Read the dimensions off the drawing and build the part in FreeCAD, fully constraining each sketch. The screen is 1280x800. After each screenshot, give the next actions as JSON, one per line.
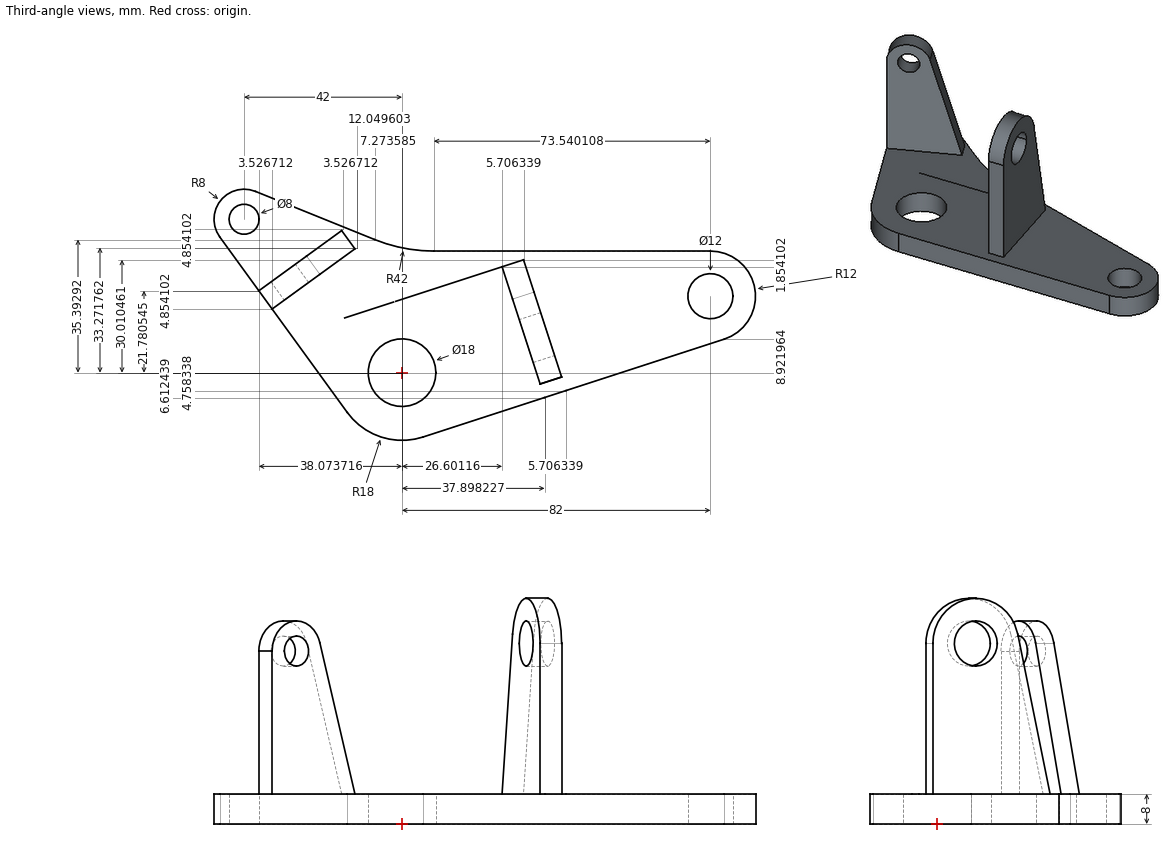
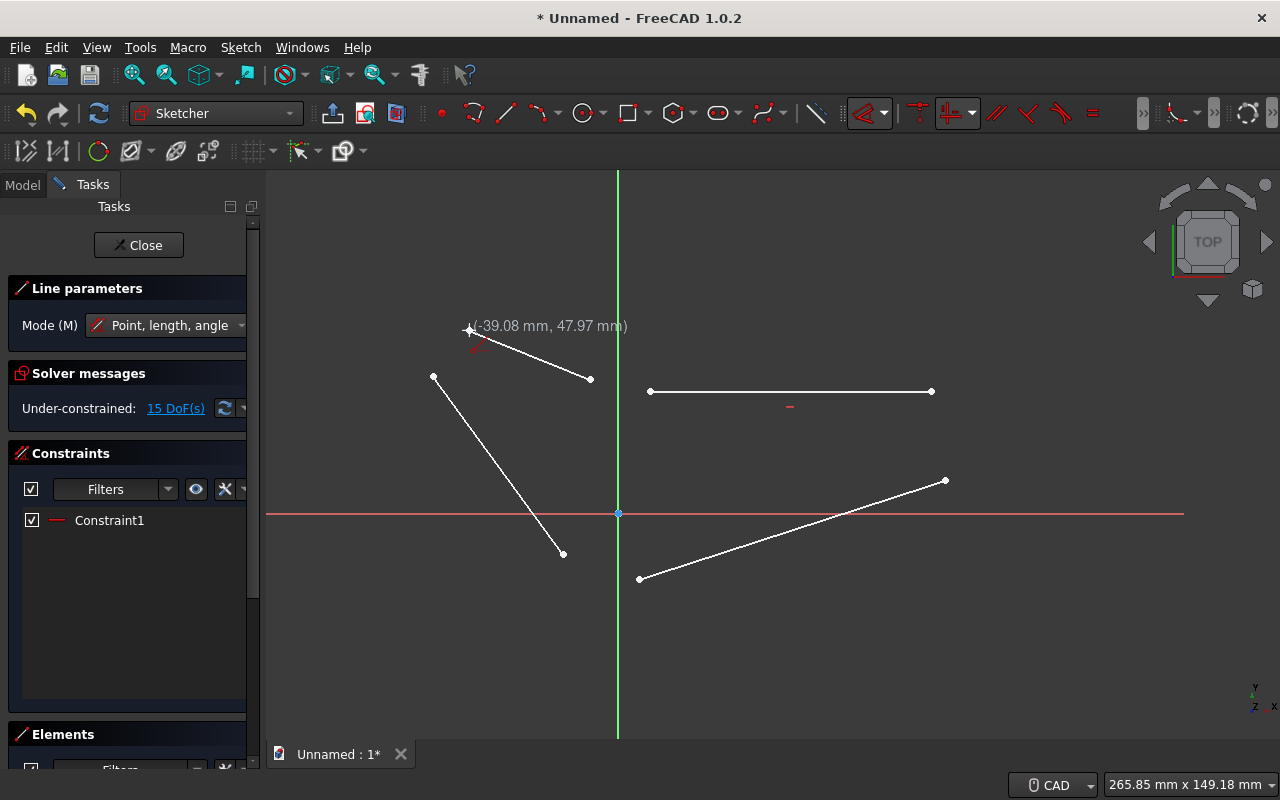
{"action": "key", "text": "g 3 a"}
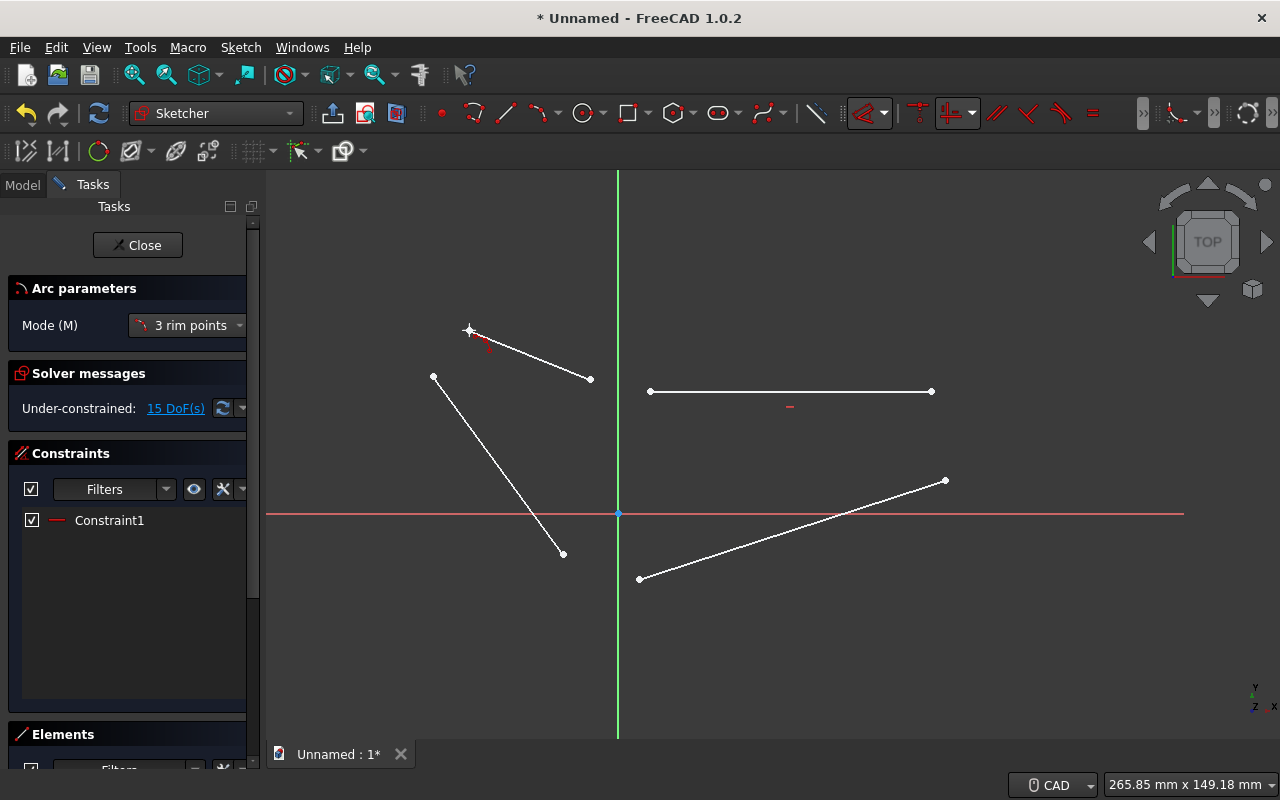
{"action": "left_click", "coordinate": [563, 555]}
{"action": "left_click", "coordinate": [639, 580]}
{"action": "left_click", "coordinate": [597, 579]}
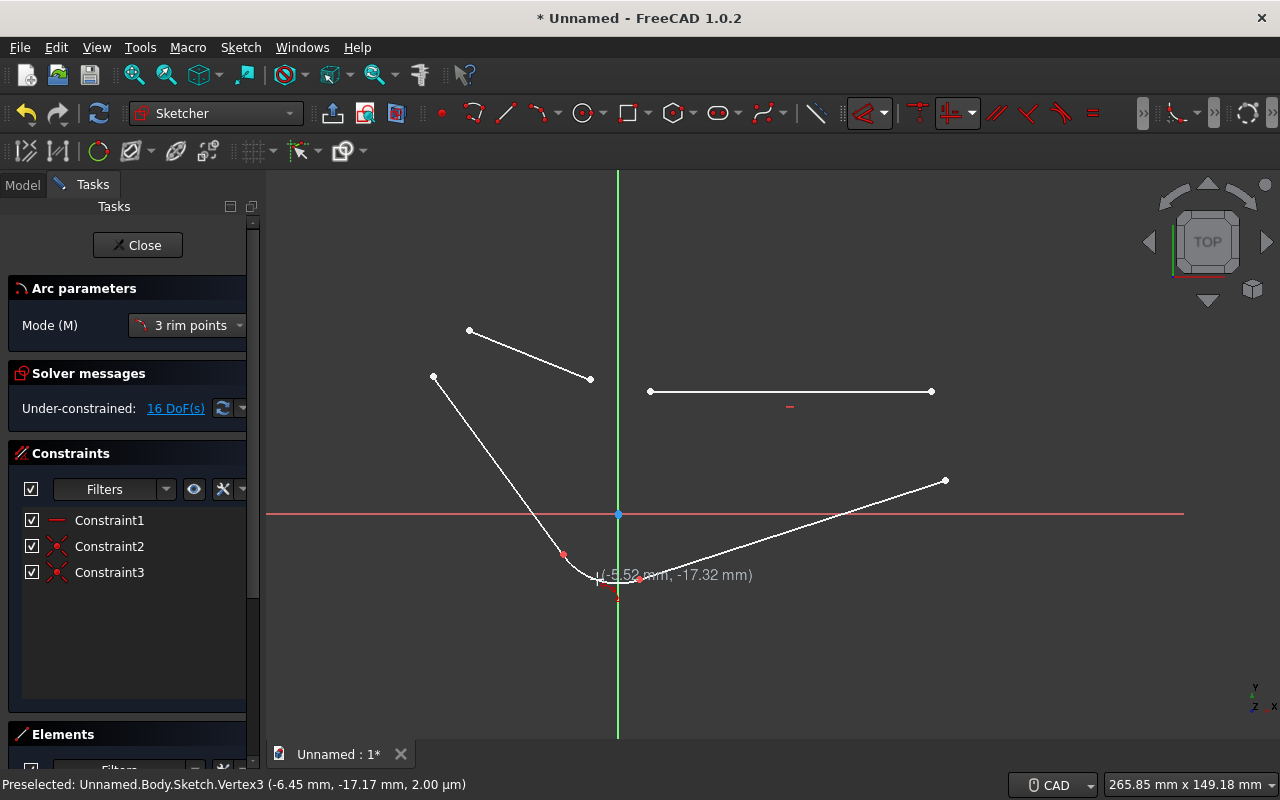
{"action": "left_click", "coordinate": [945, 481]}
{"action": "left_click", "coordinate": [931, 392]}
{"action": "left_click", "coordinate": [976, 429]}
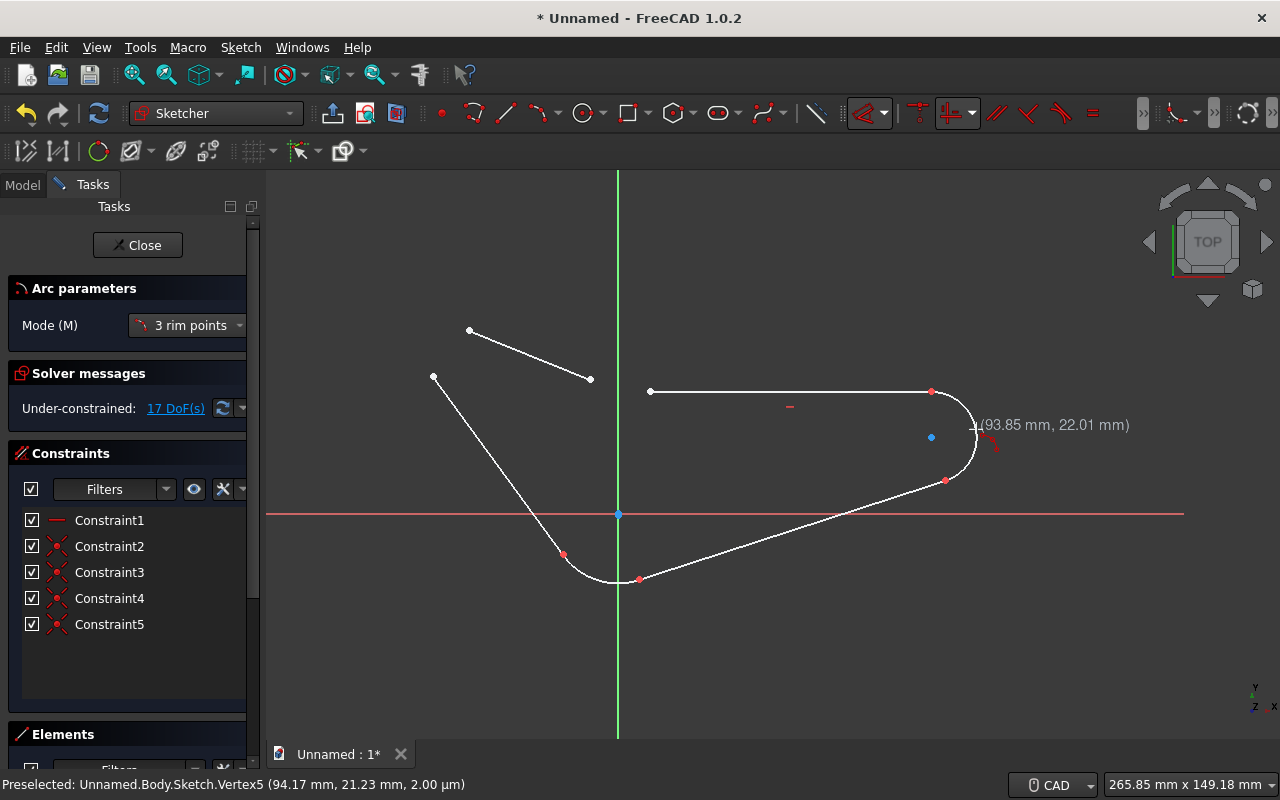
{"action": "left_click", "coordinate": [650, 392]}
{"action": "left_click", "coordinate": [590, 380]}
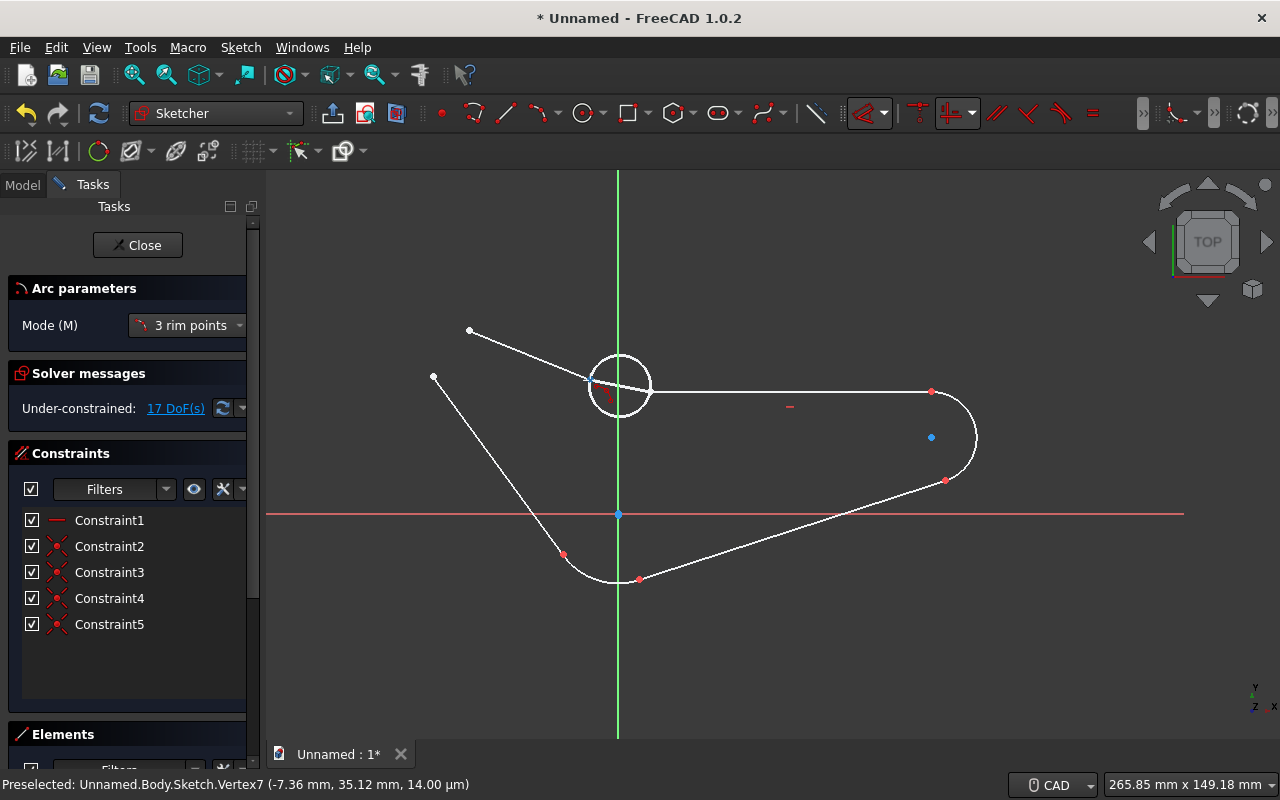
{"action": "scroll", "coordinate": [626, 389], "scroll_direction": "up", "scroll_amount": 9}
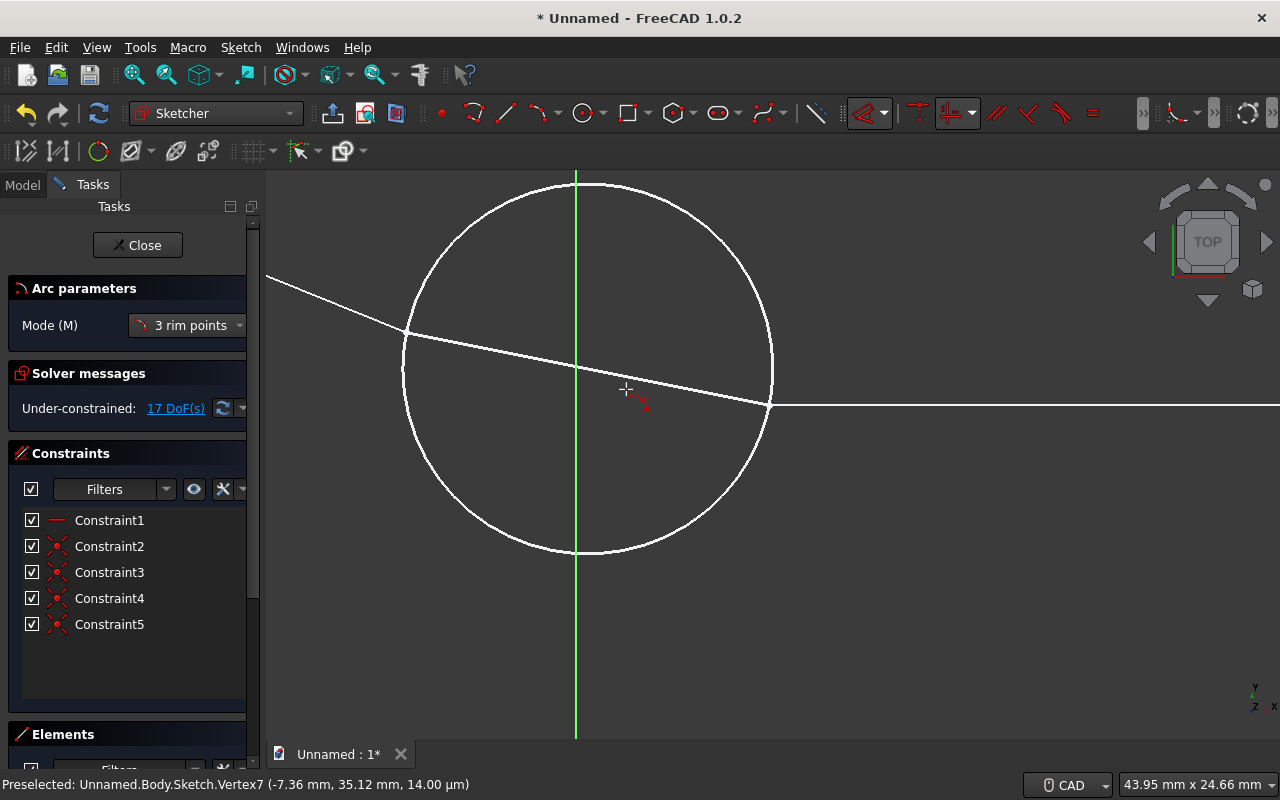
{"action": "left_click", "coordinate": [623, 385]}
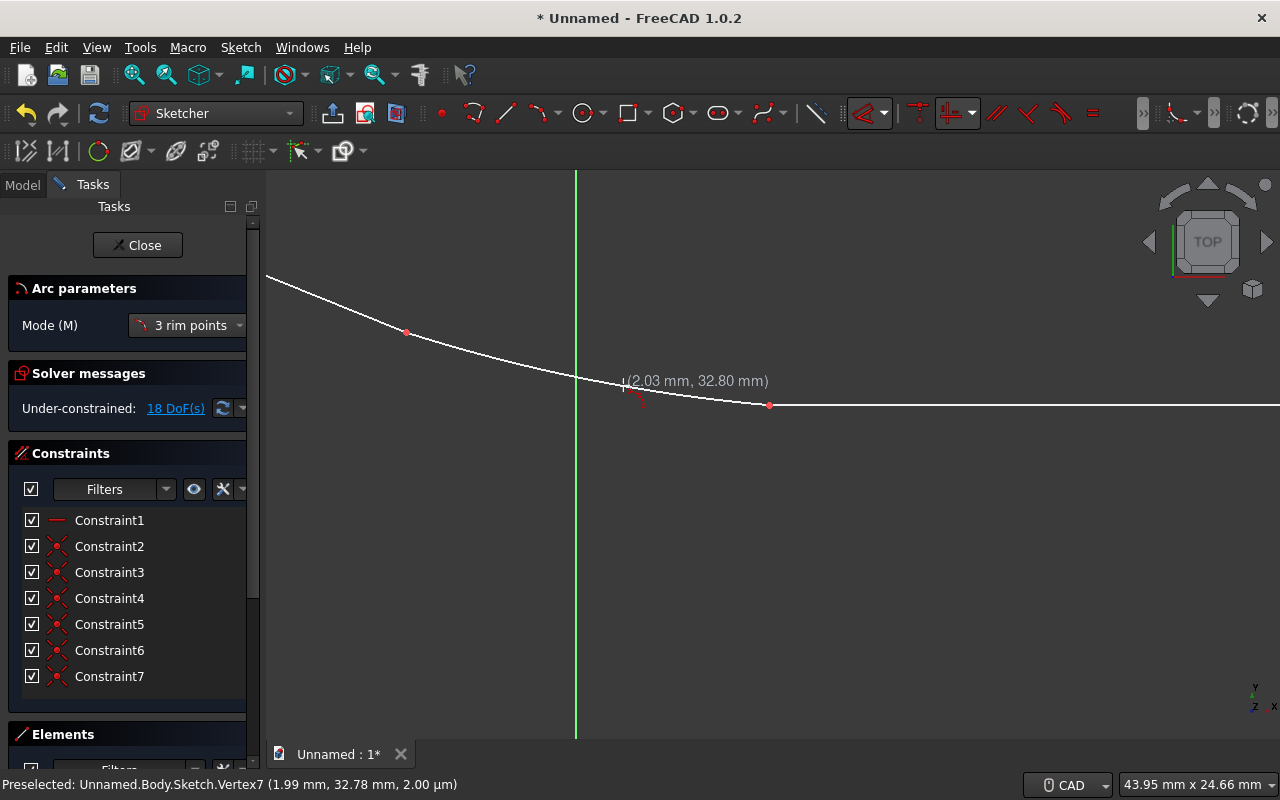
{"action": "scroll", "coordinate": [626, 389], "scroll_direction": "down", "scroll_amount": 9}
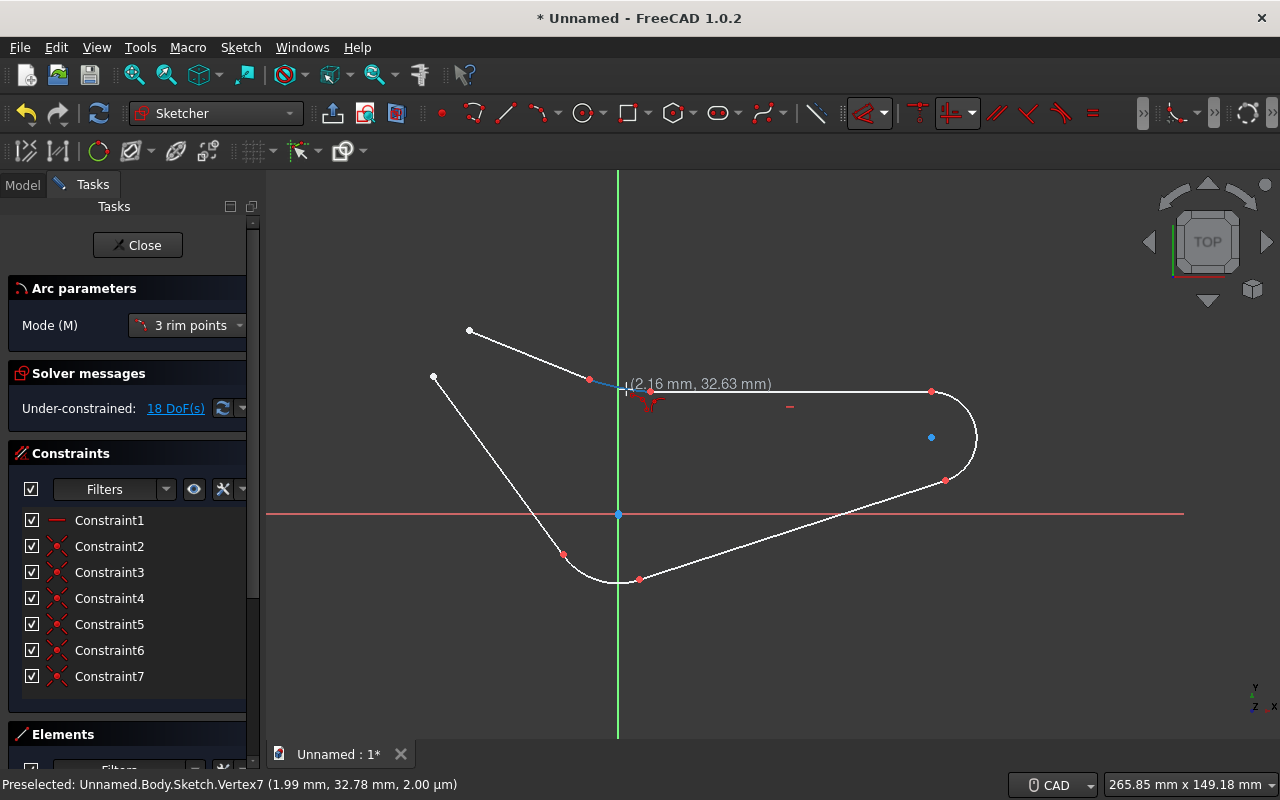
{"action": "left_click", "coordinate": [469, 331]}
{"action": "left_click", "coordinate": [433, 377]}
{"action": "left_click", "coordinate": [434, 340]}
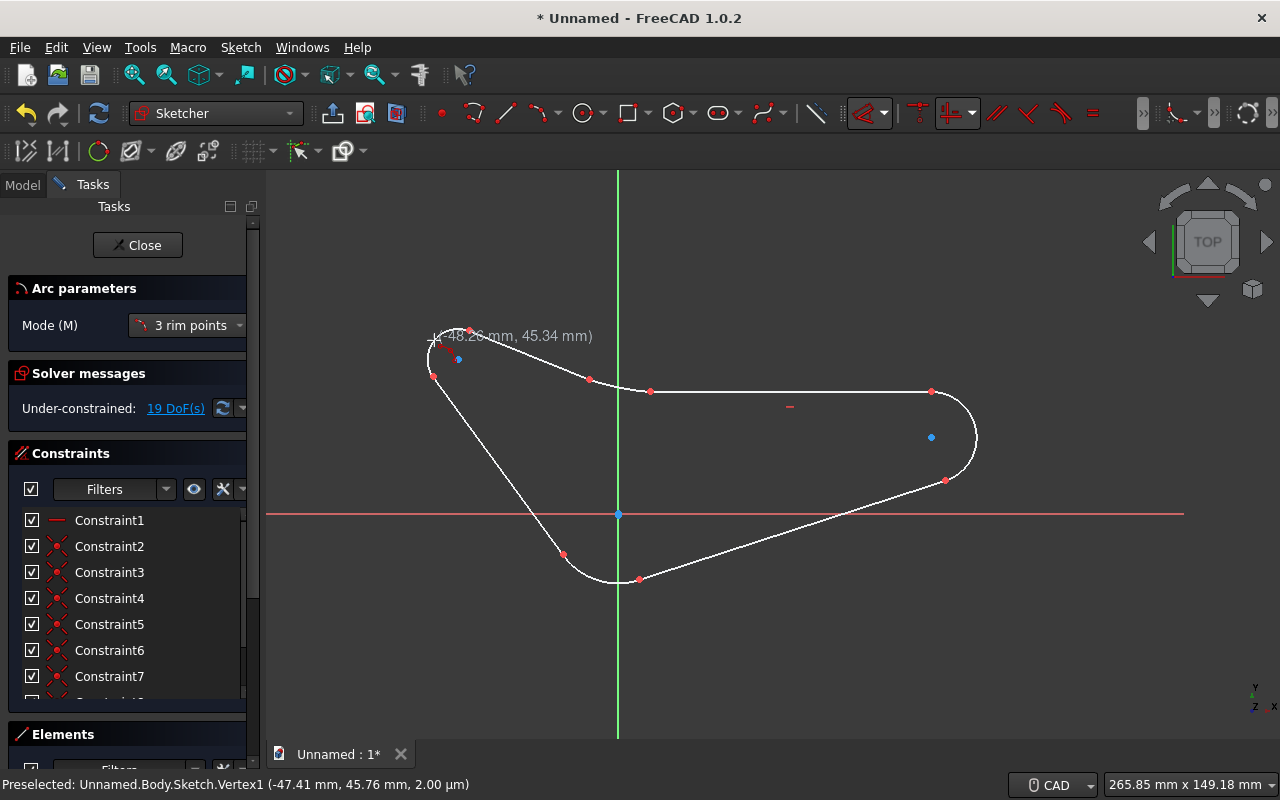
{"action": "key", "text": "g c"}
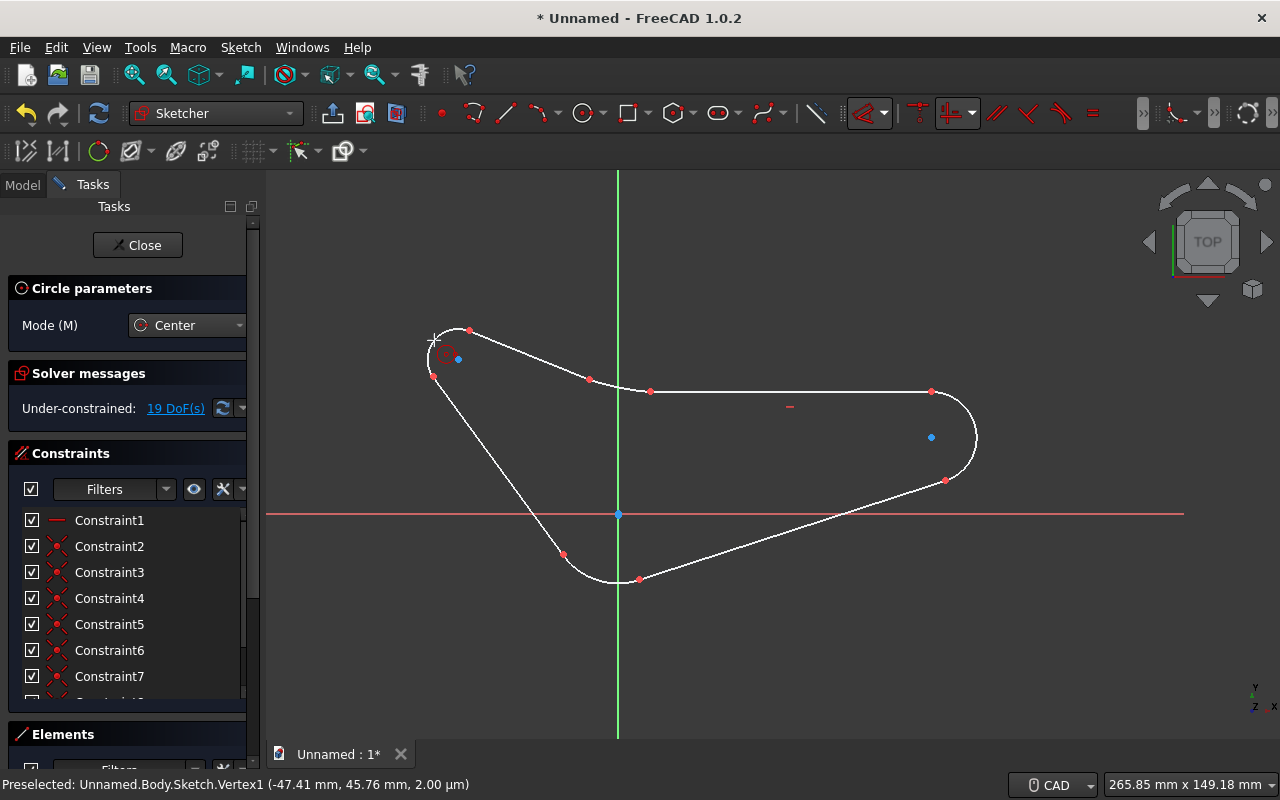
{"action": "left_click", "coordinate": [618, 514]}
{"action": "left_click", "coordinate": [642, 490]}